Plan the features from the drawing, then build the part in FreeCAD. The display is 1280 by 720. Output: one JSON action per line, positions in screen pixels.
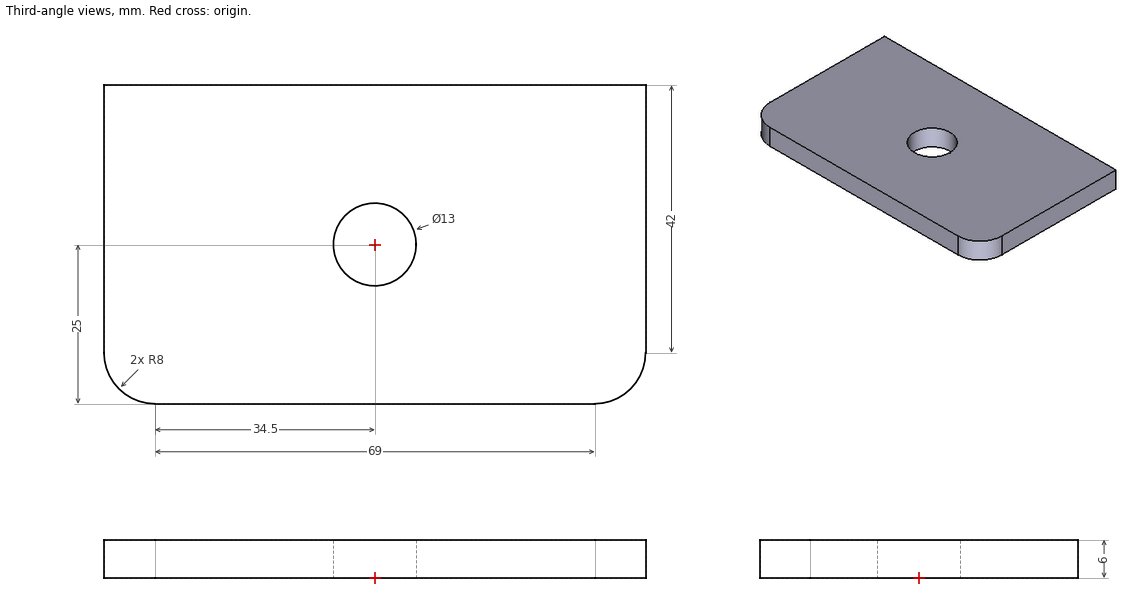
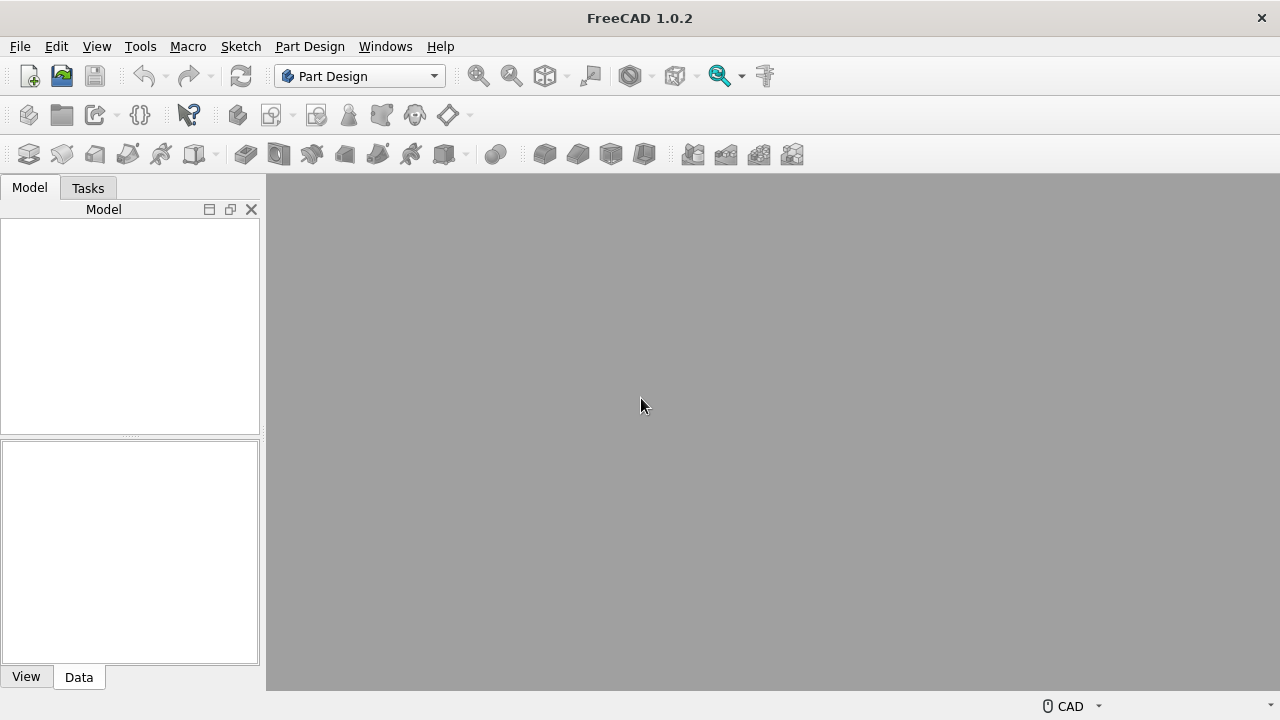
{"action": "left_click", "coordinate": [29, 76]}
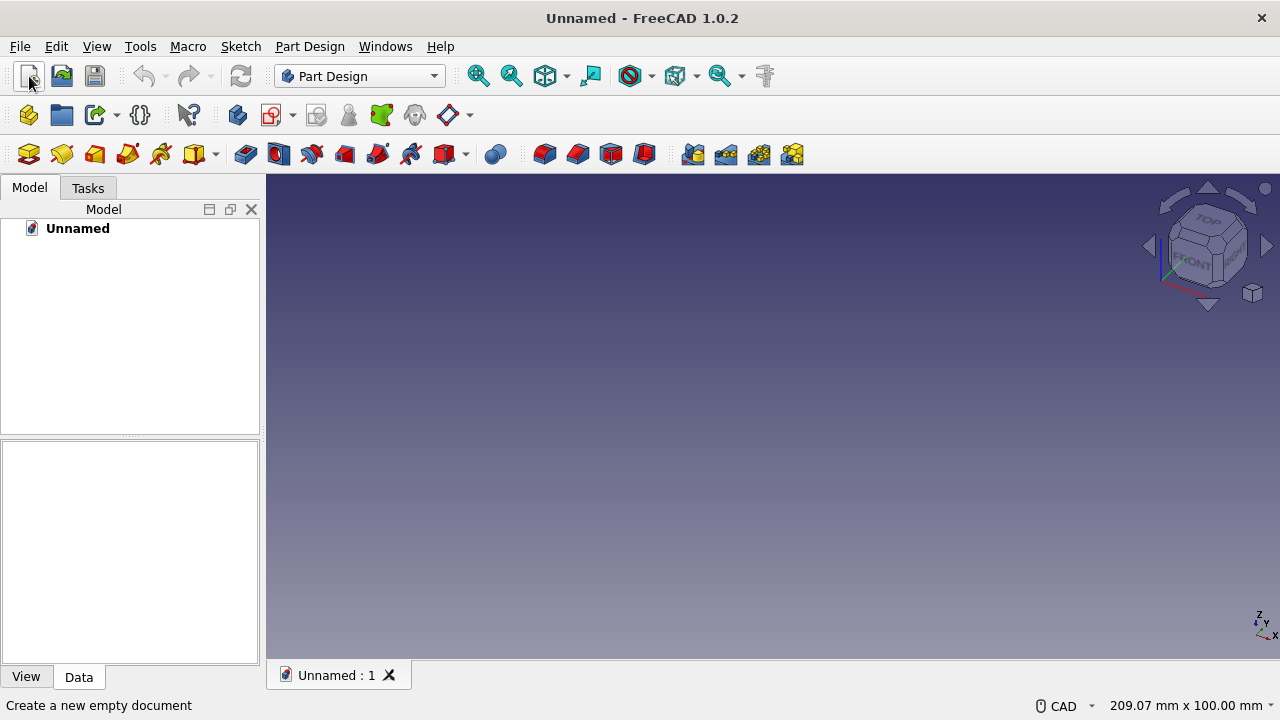
{"action": "left_click", "coordinate": [270, 116]}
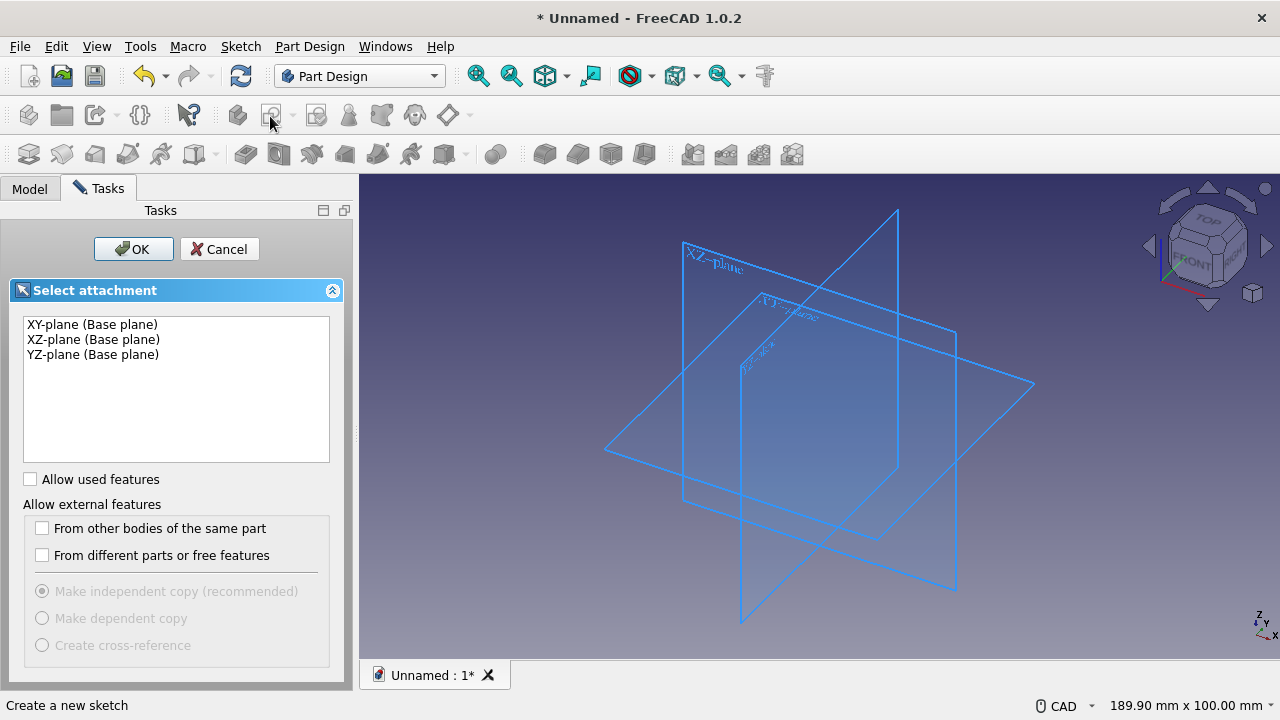
{"action": "left_click", "coordinate": [84, 324]}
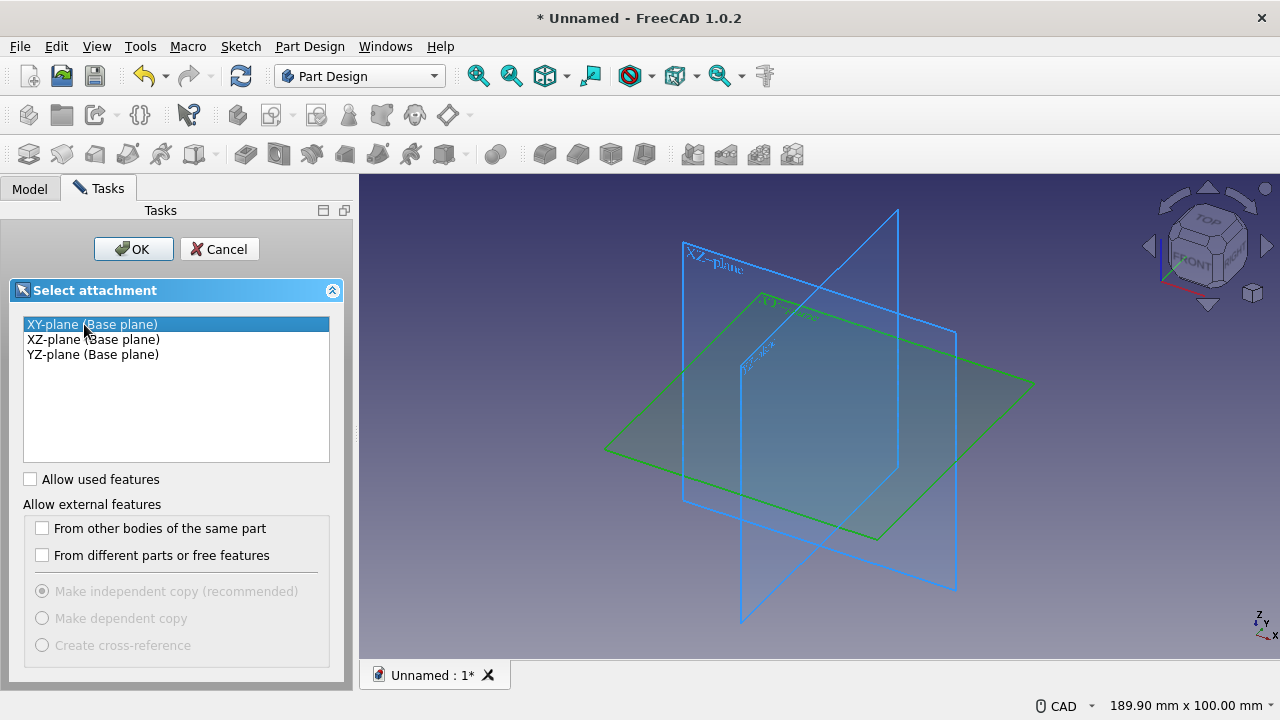
{"action": "left_click", "coordinate": [134, 249]}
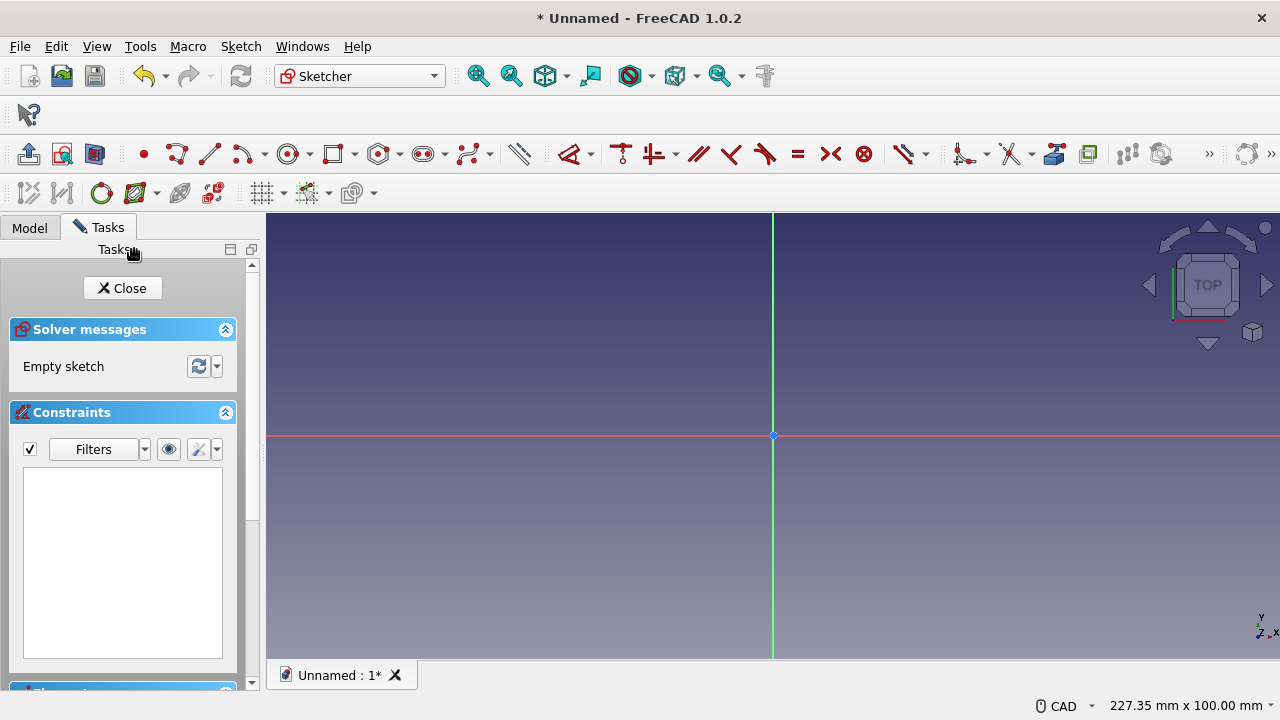
{"action": "left_click", "coordinate": [210, 154]}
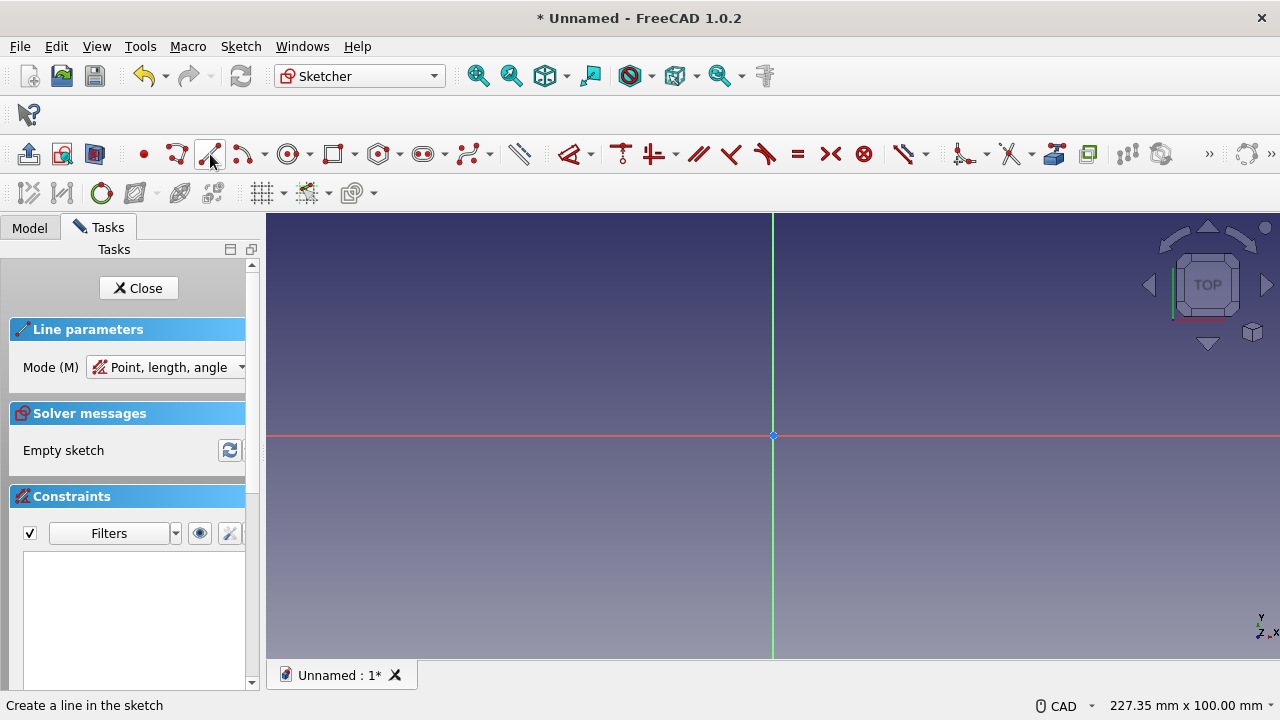
{"action": "left_click", "coordinate": [619, 548]}
{"action": "left_click", "coordinate": [927, 548]}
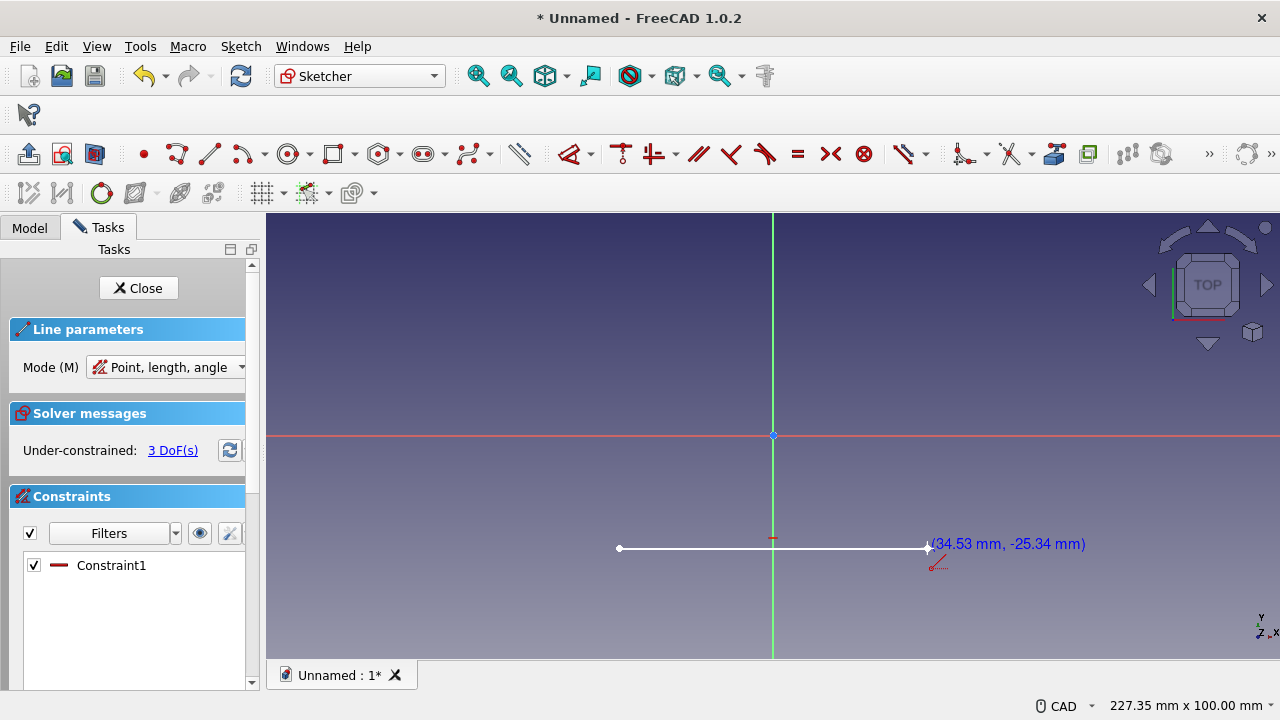
{"action": "left_click", "coordinate": [177, 154]}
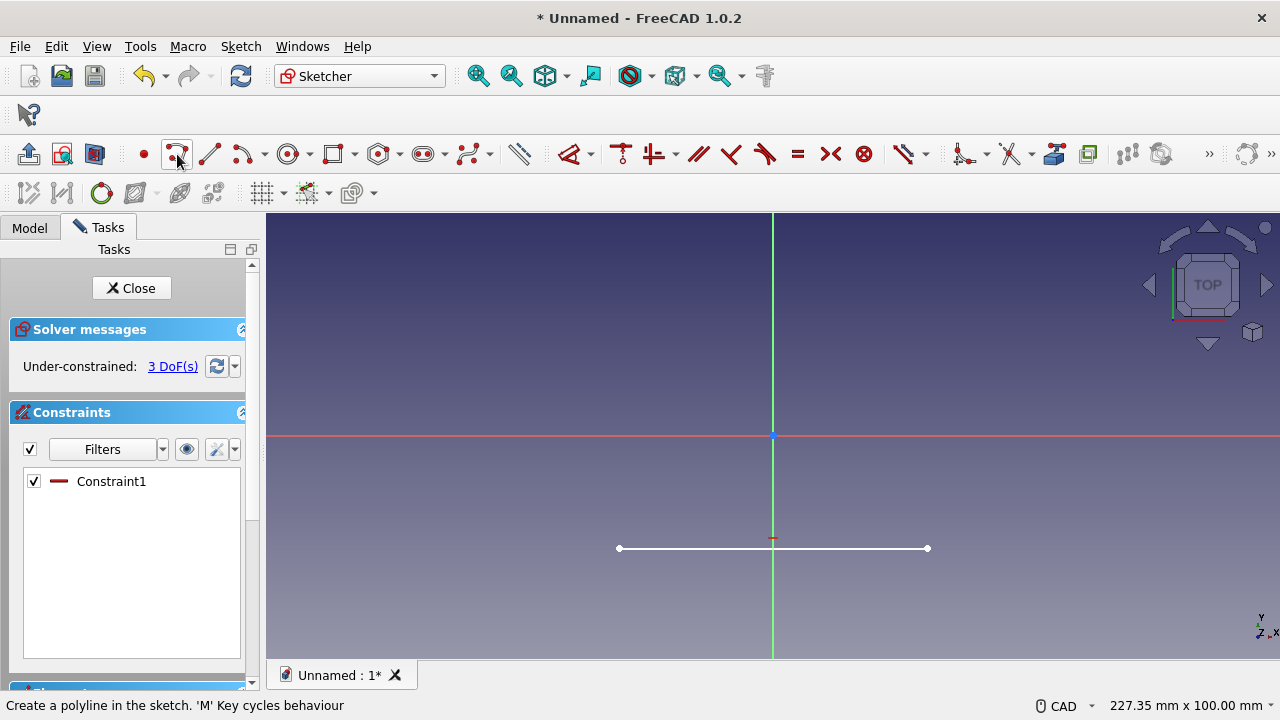
{"action": "left_click", "coordinate": [963, 512]}
{"action": "left_click", "coordinate": [963, 324]}
{"action": "left_click", "coordinate": [583, 324]}
{"action": "left_click", "coordinate": [583, 512]}
{"action": "right_click", "coordinate": [583, 512]}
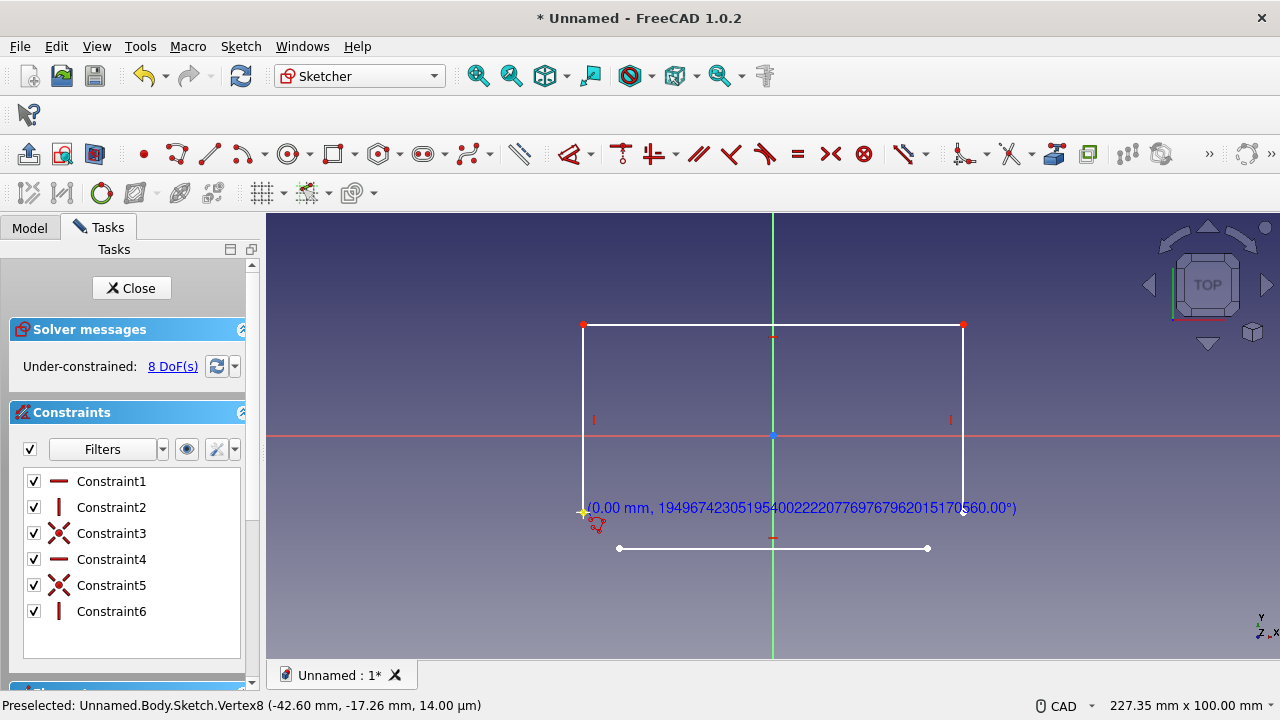
{"action": "left_click", "coordinate": [264, 154]}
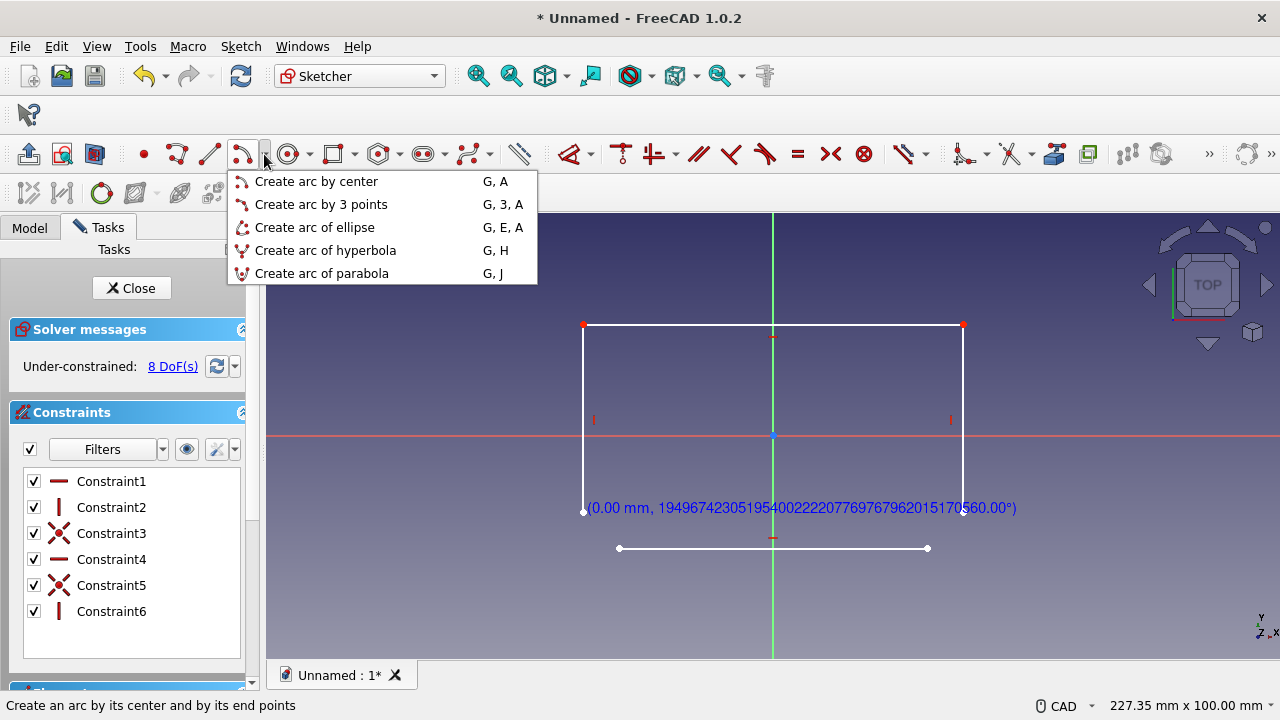
{"action": "left_click", "coordinate": [382, 204]}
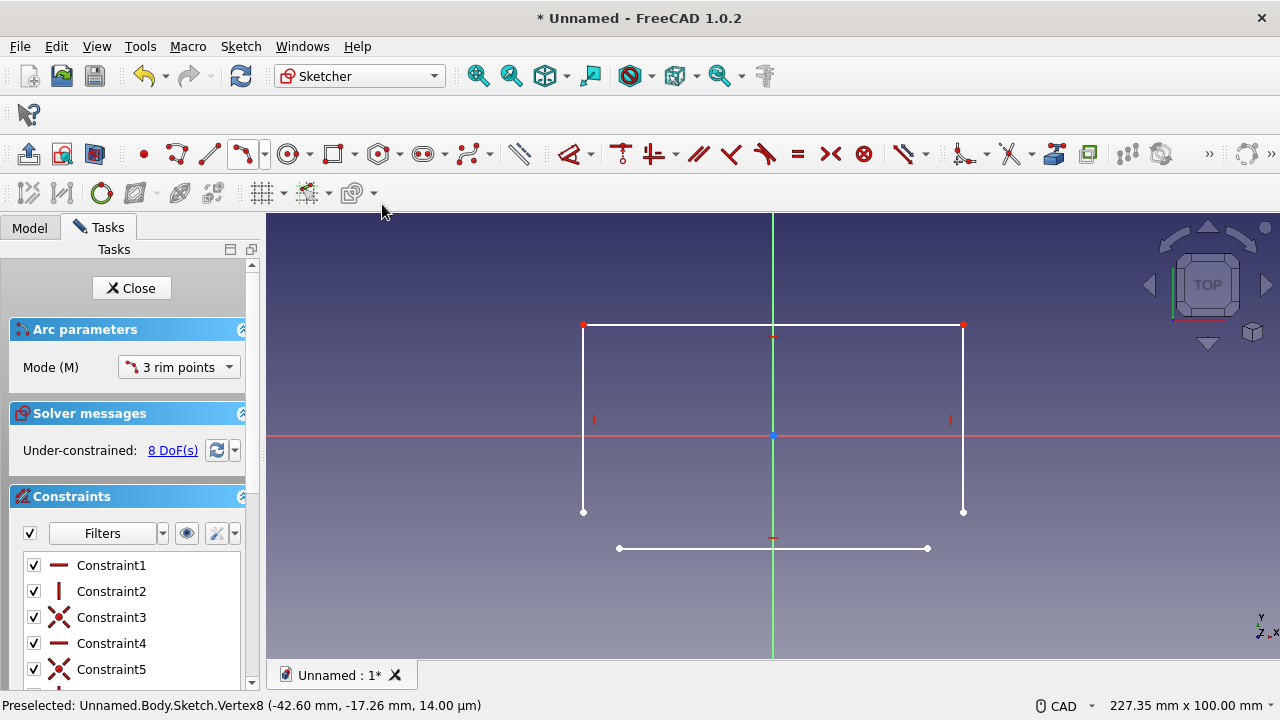
{"action": "left_click", "coordinate": [927, 549]}
{"action": "left_click", "coordinate": [963, 513]}